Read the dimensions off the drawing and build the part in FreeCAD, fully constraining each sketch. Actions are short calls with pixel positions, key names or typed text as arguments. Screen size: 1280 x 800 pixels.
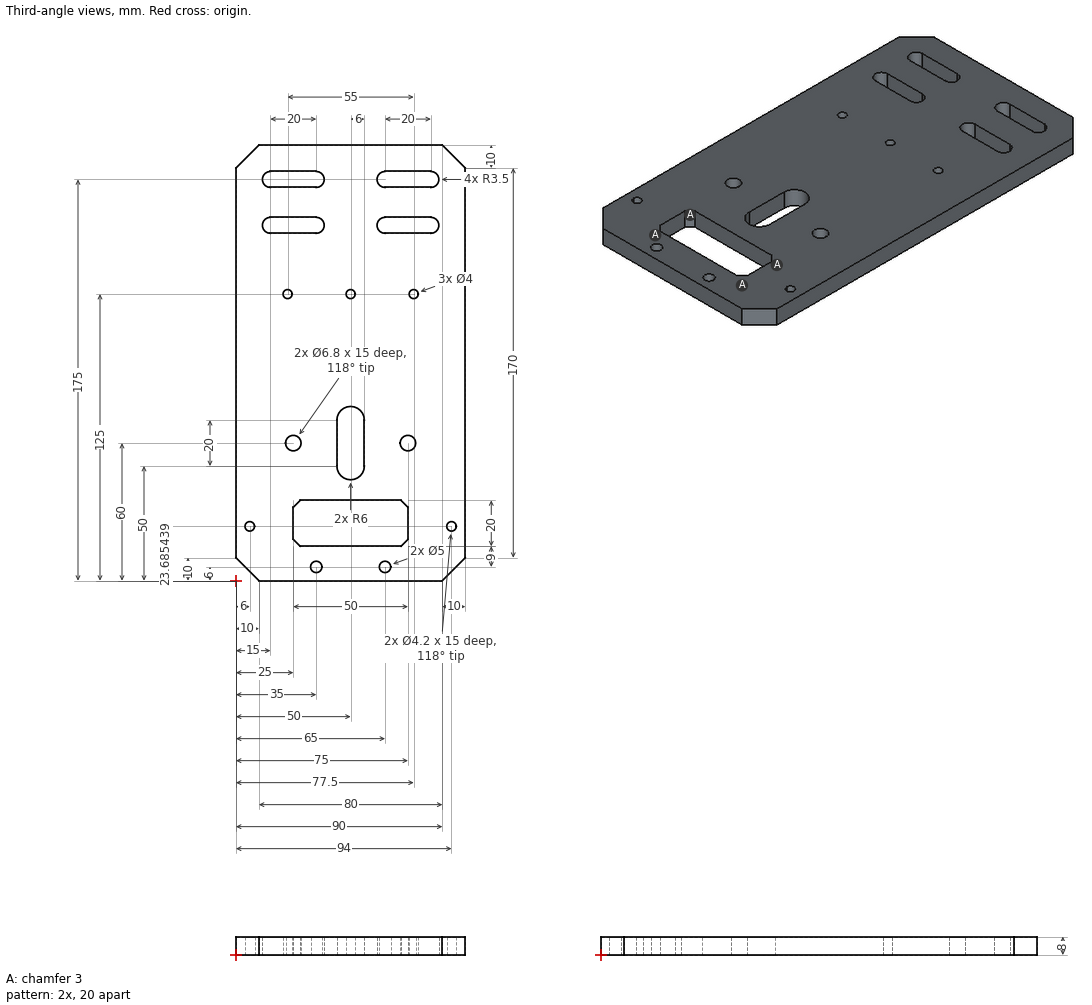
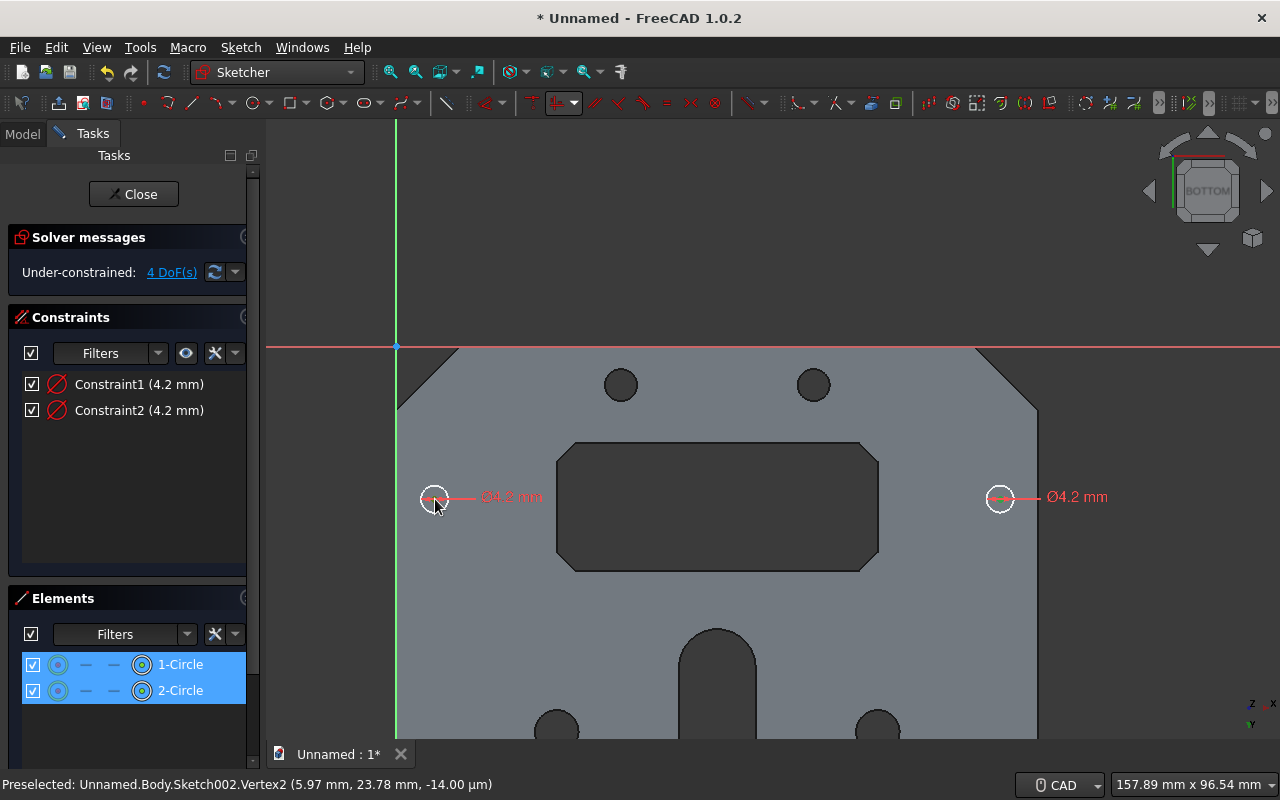
click(576, 104)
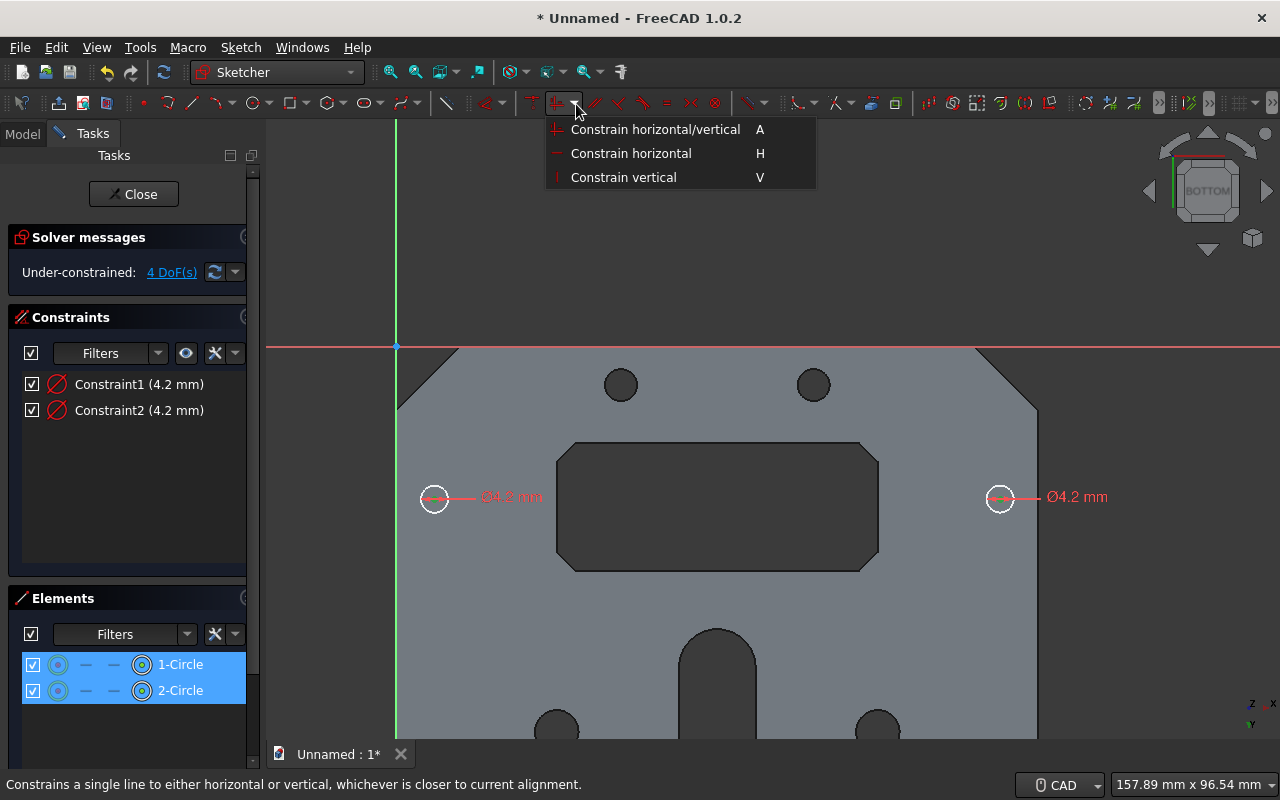
click(681, 153)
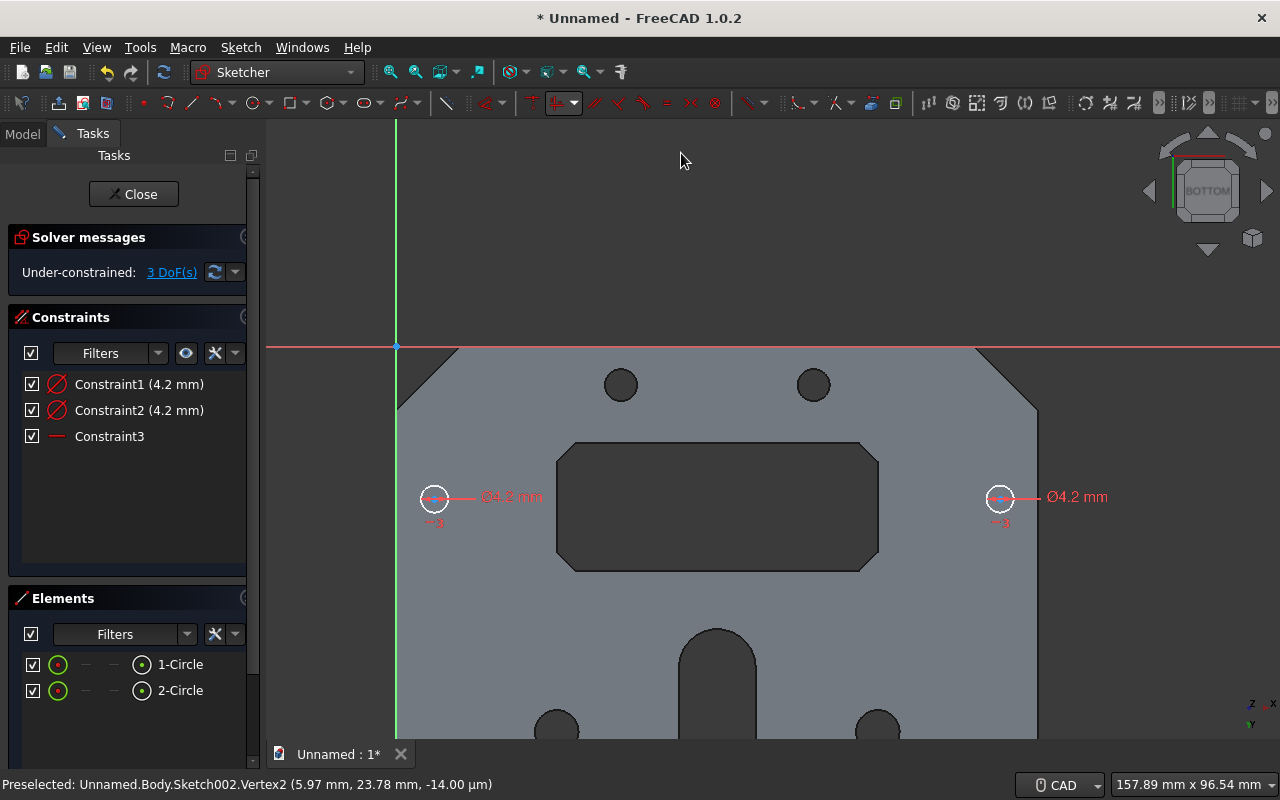
click(486, 104)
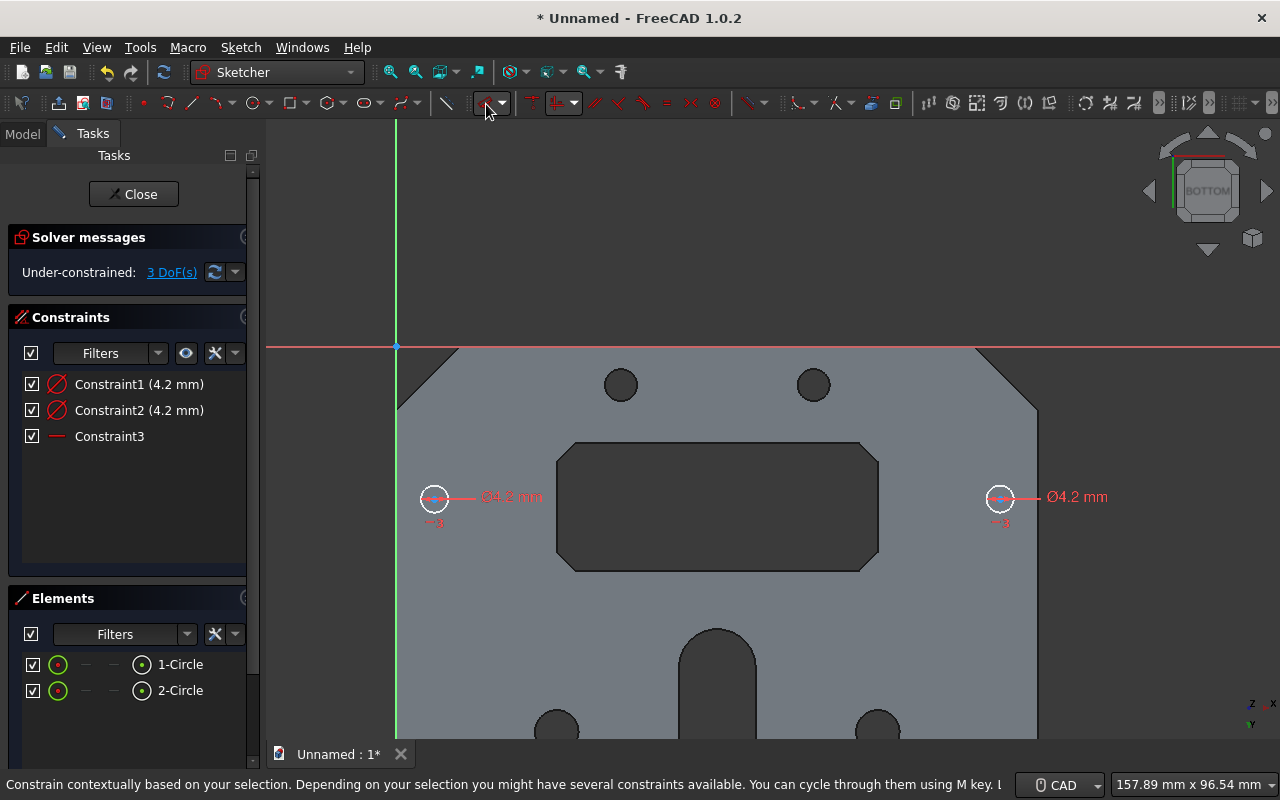
click(435, 499)
click(415, 313)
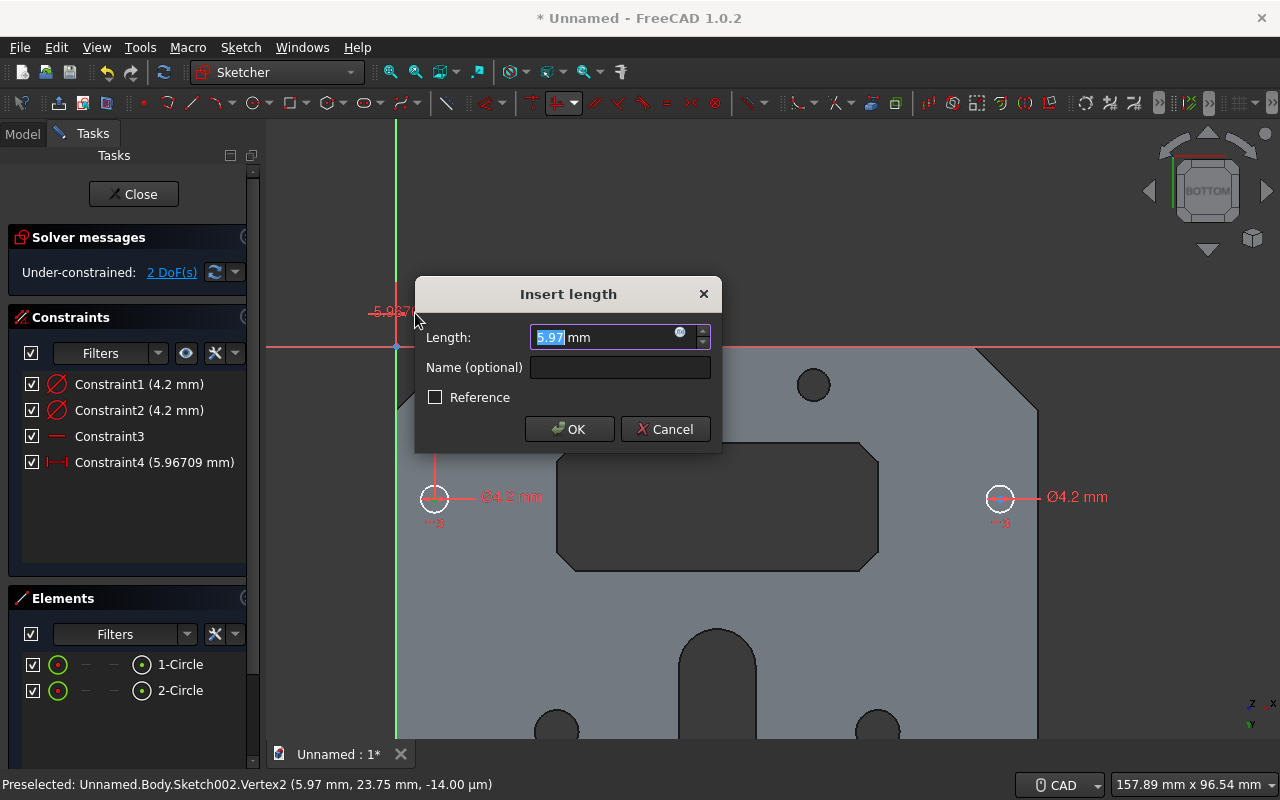
text(6)
key(Return)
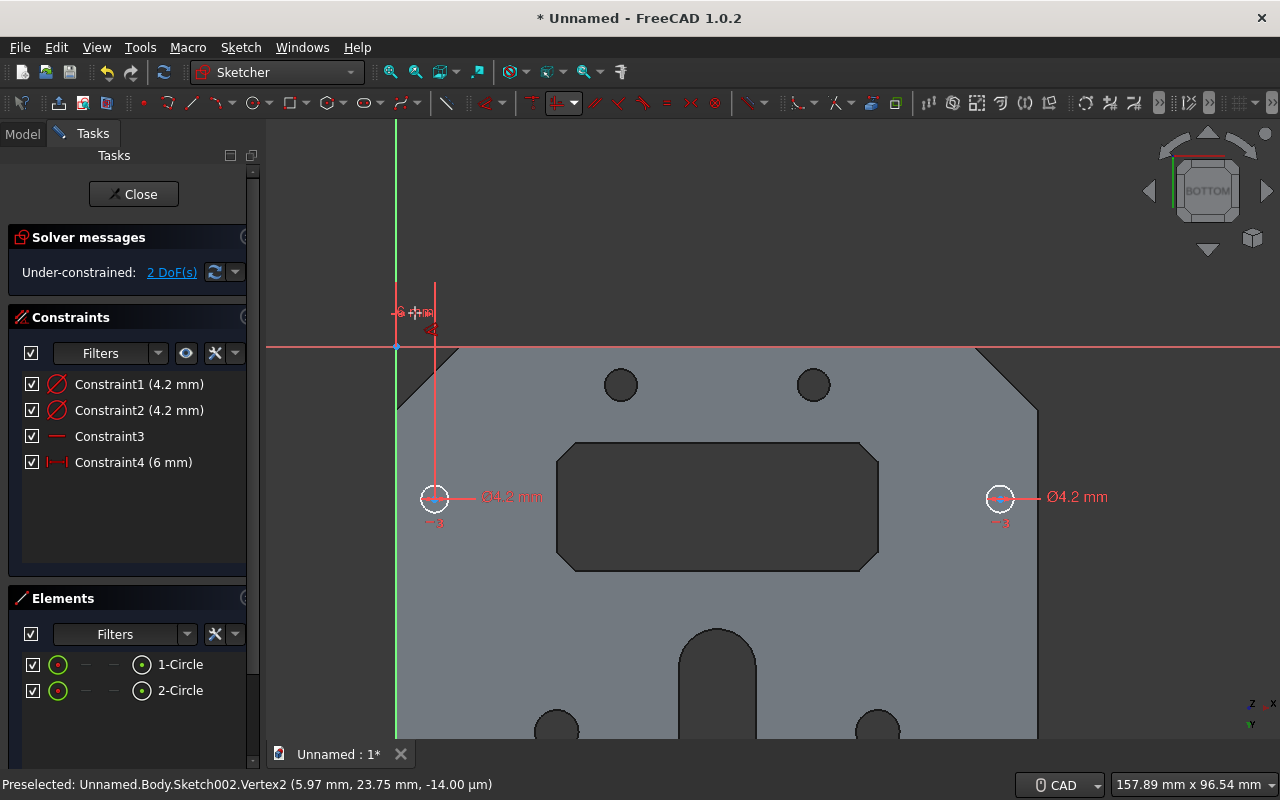
click(1000, 499)
click(698, 313)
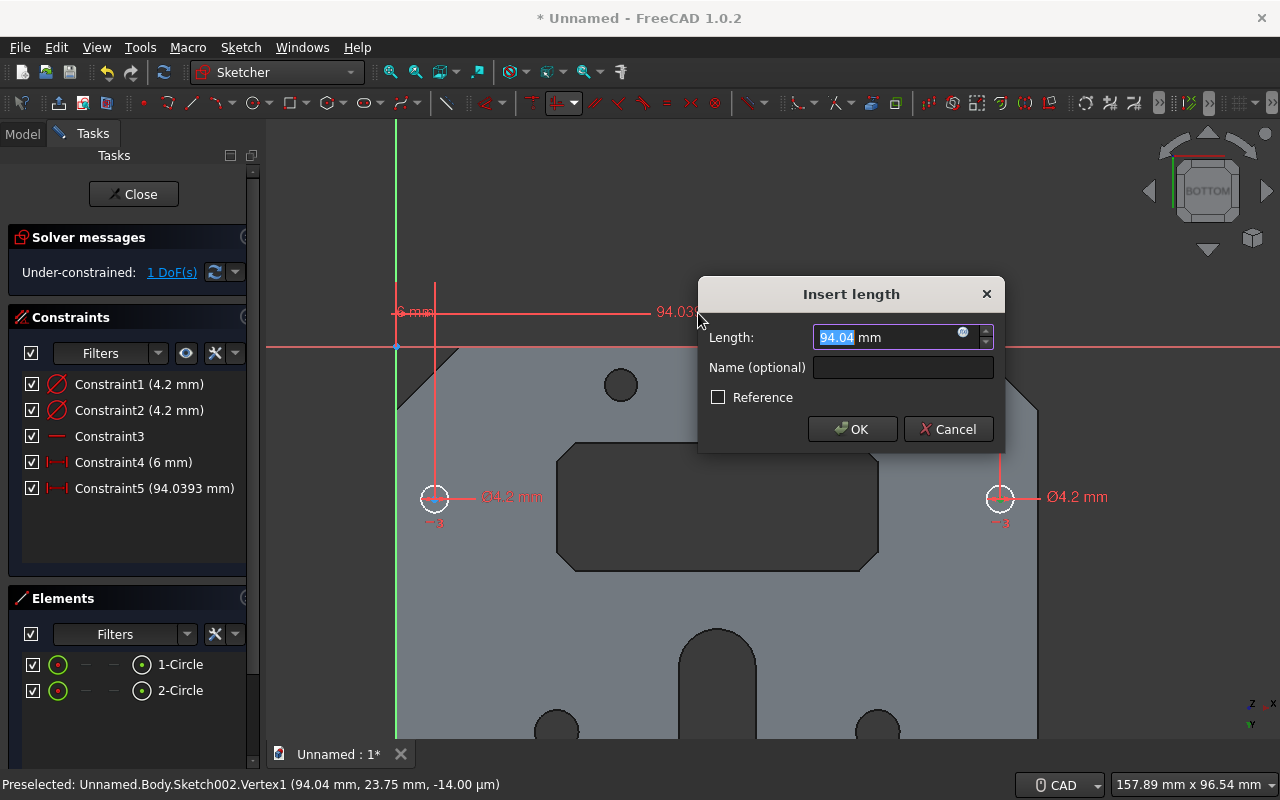
text(94)
key(Return)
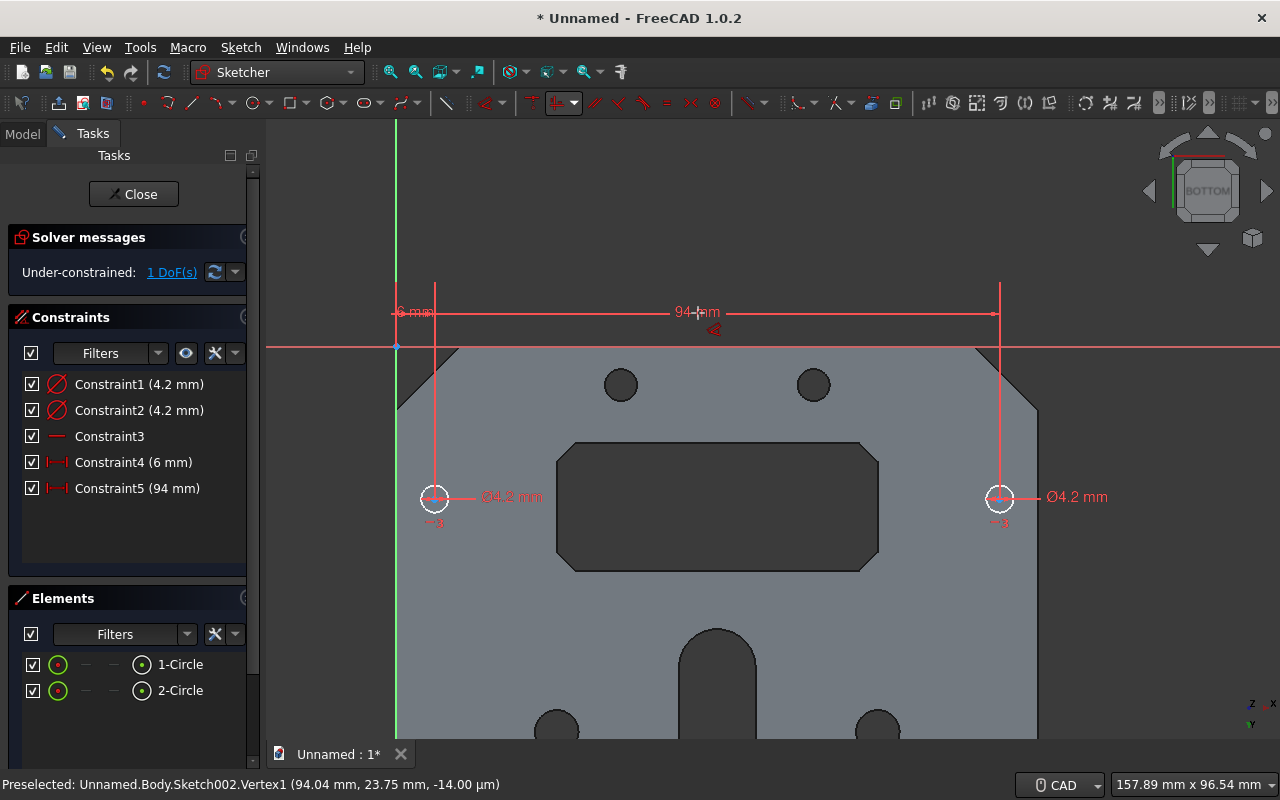
click(1000, 499)
click(362, 423)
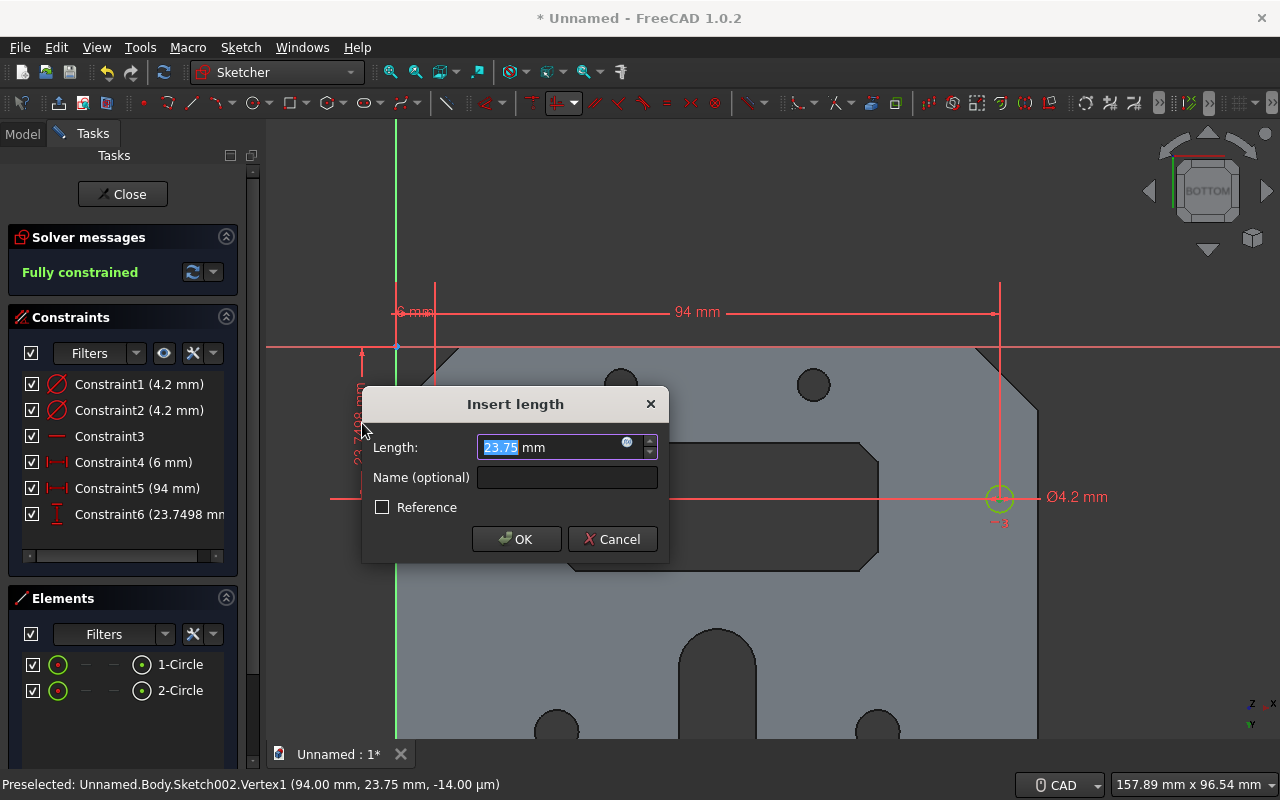
text(23.685439)
key(Return)
key(Escape)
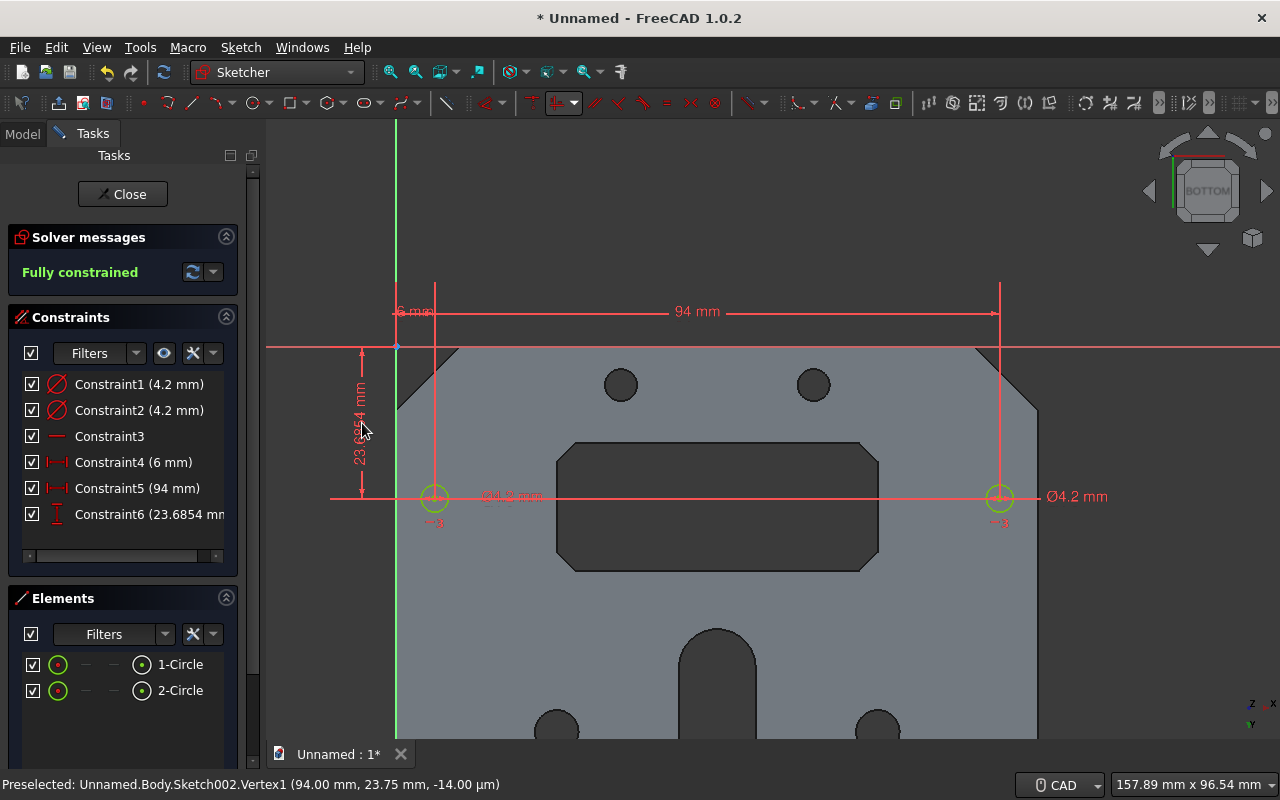
click(123, 194)